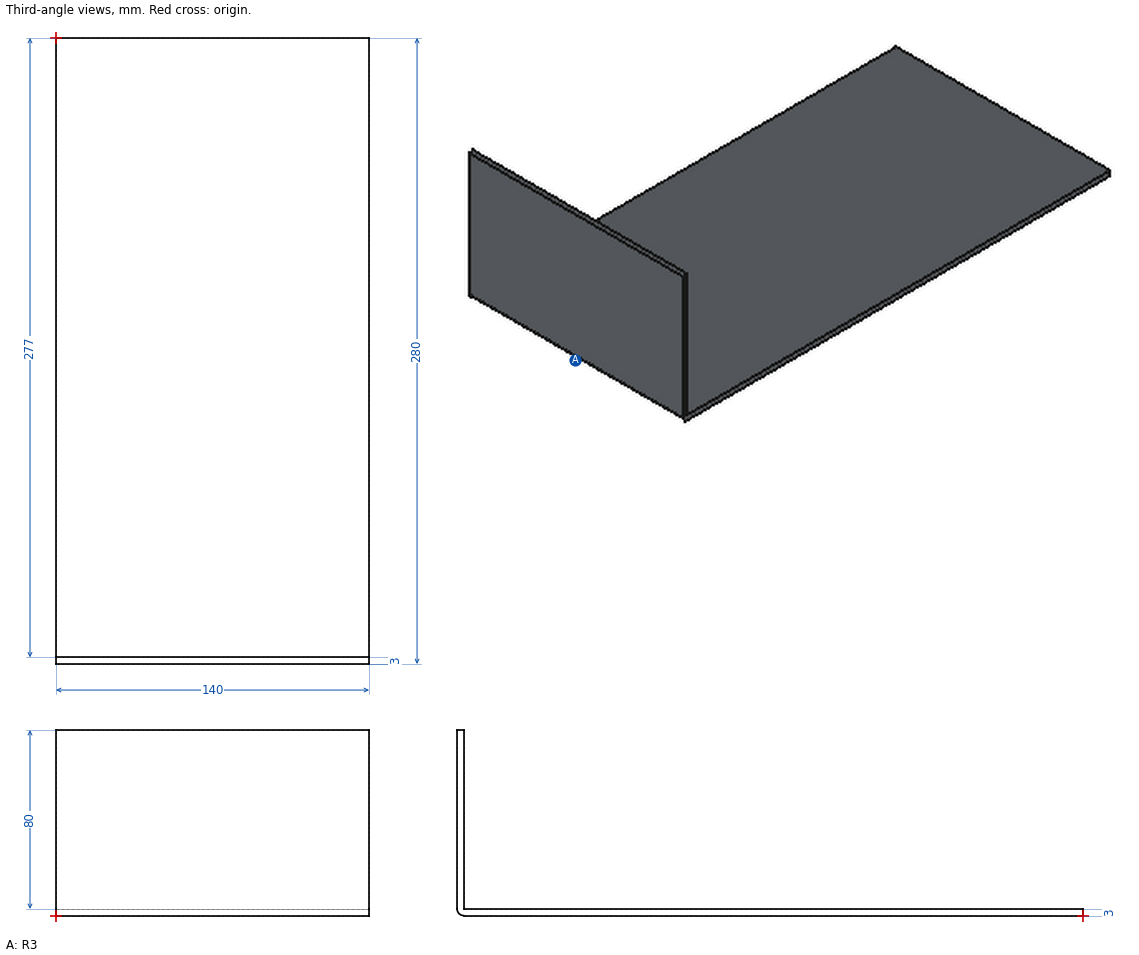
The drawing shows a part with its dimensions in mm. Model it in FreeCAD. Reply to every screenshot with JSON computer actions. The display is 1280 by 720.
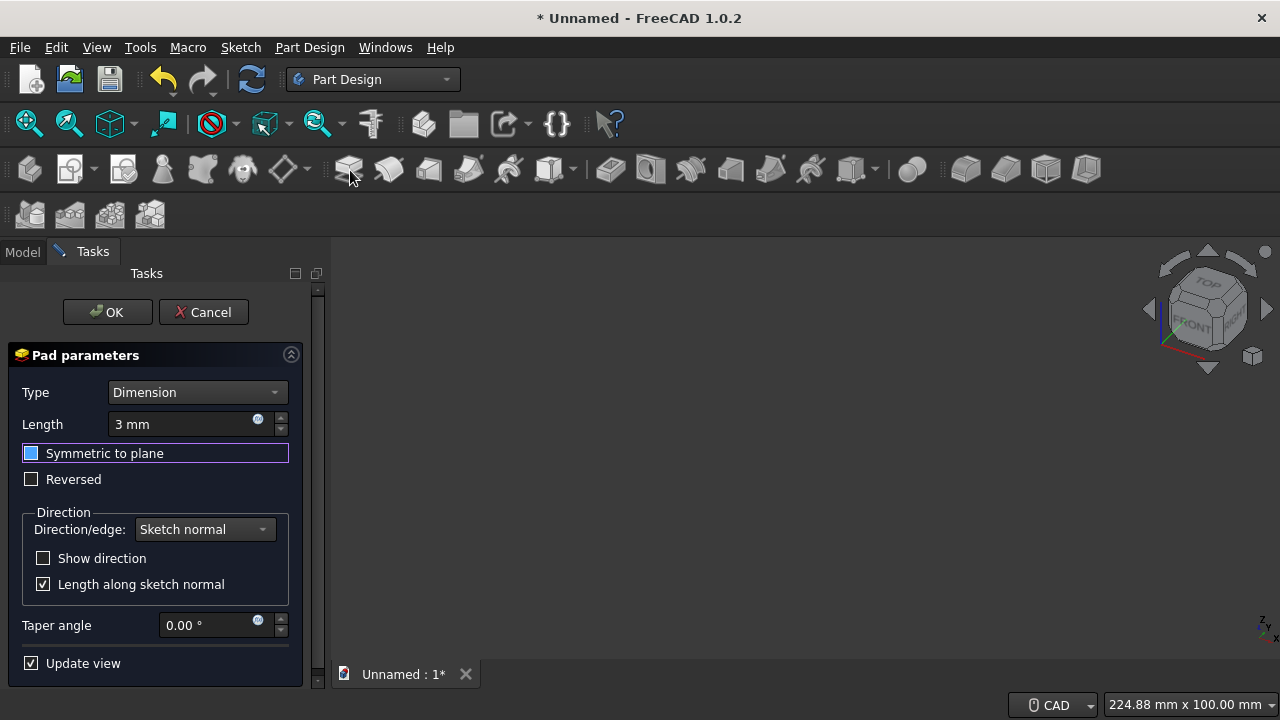
{"action": "left_click", "coordinate": [108, 312]}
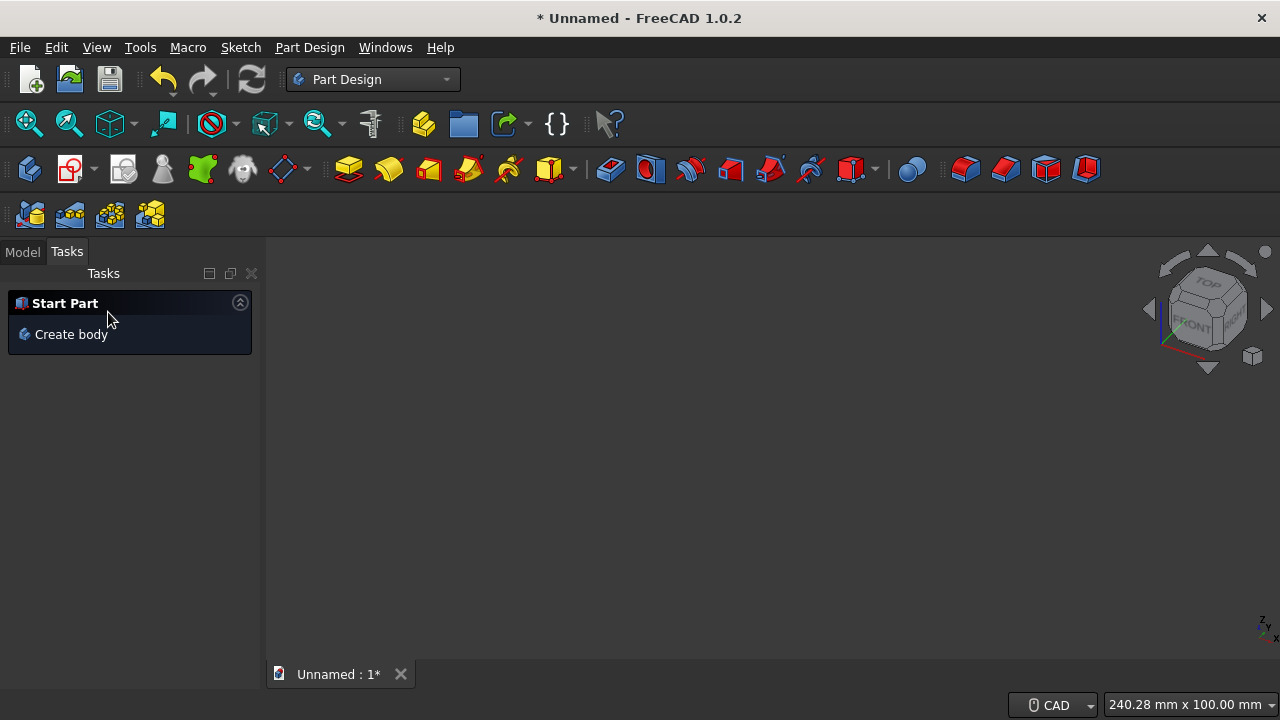
{"action": "key", "text": "v f"}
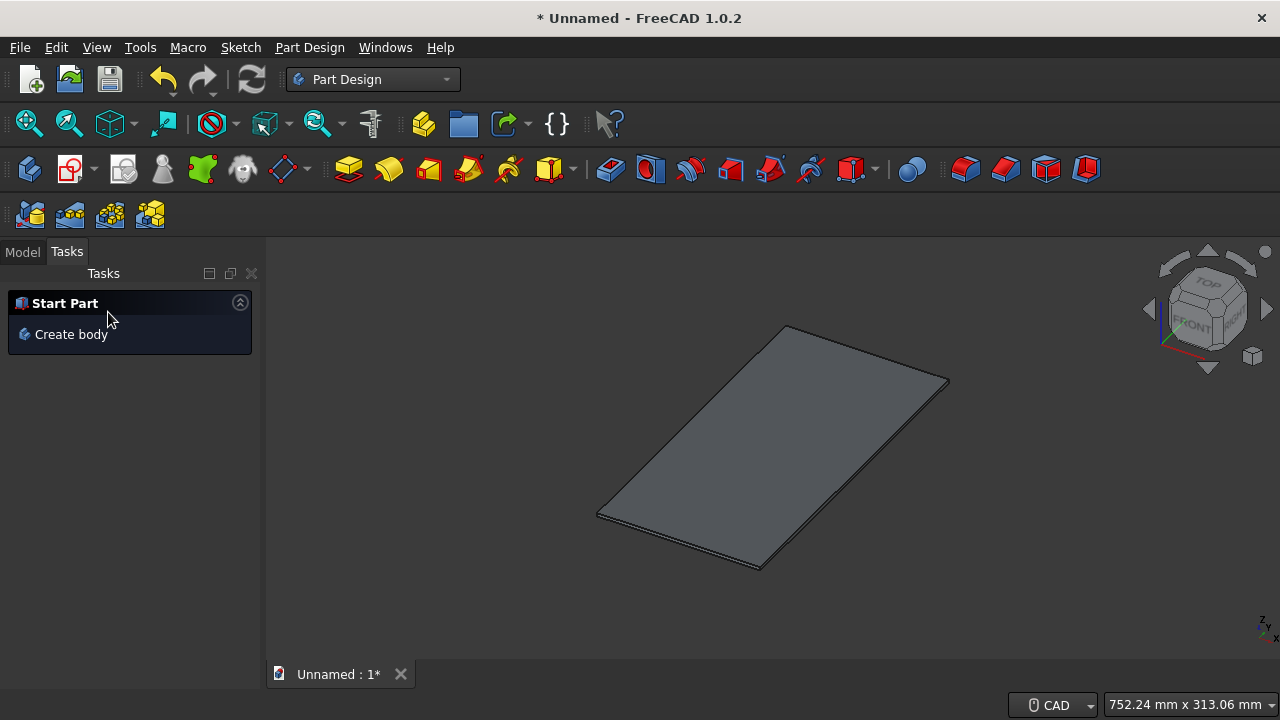
{"action": "left_click", "coordinate": [800, 419]}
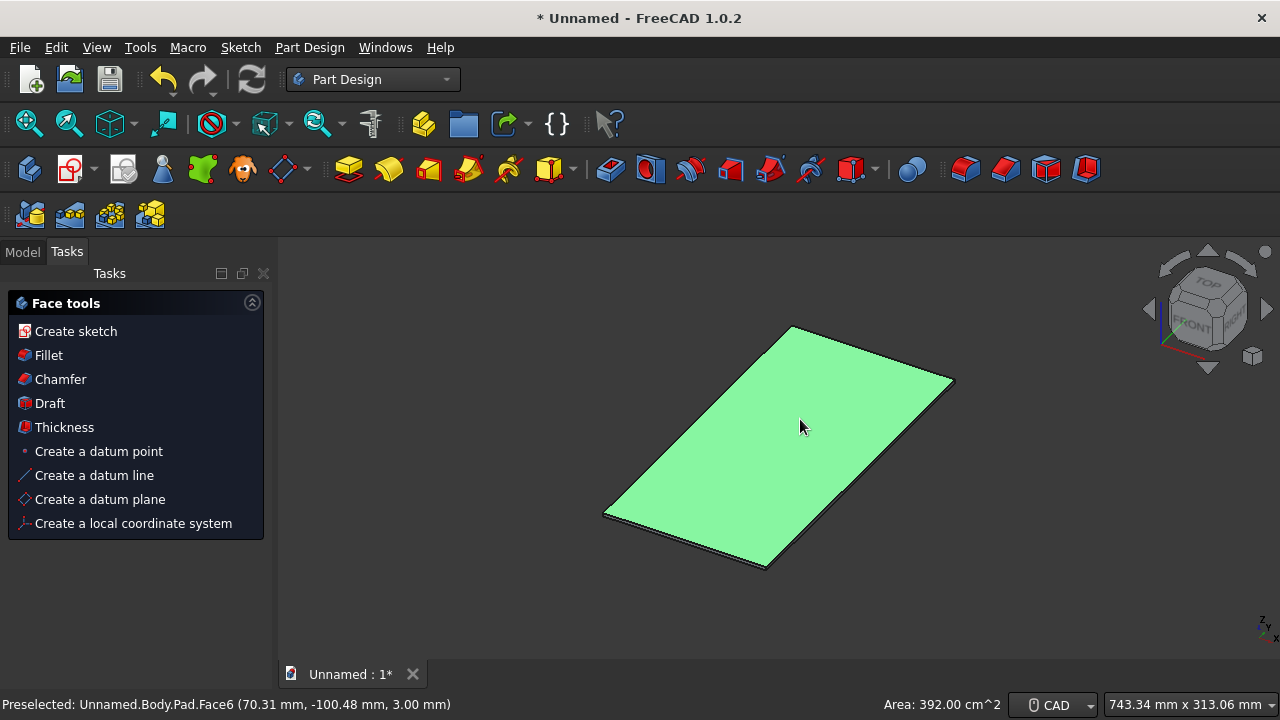
{"action": "left_click", "coordinate": [70, 170]}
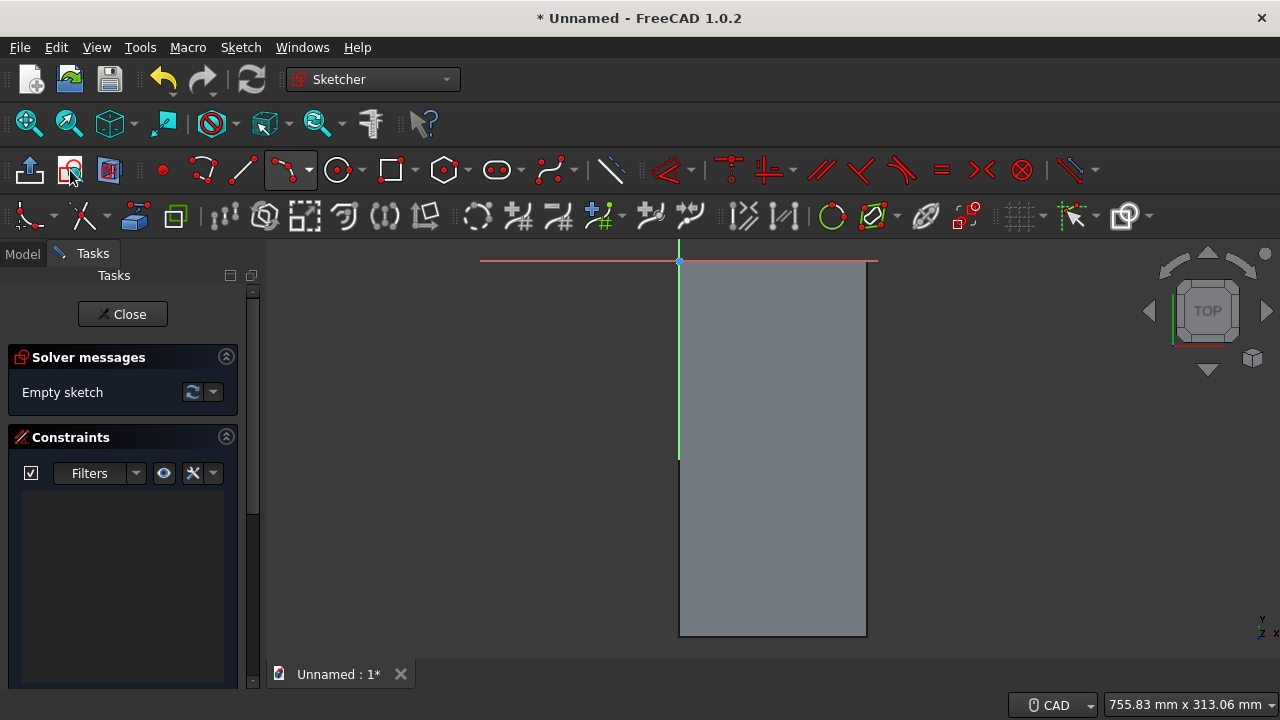
{"action": "scroll", "coordinate": [565, 449], "scroll_direction": "down", "scroll_amount": 2}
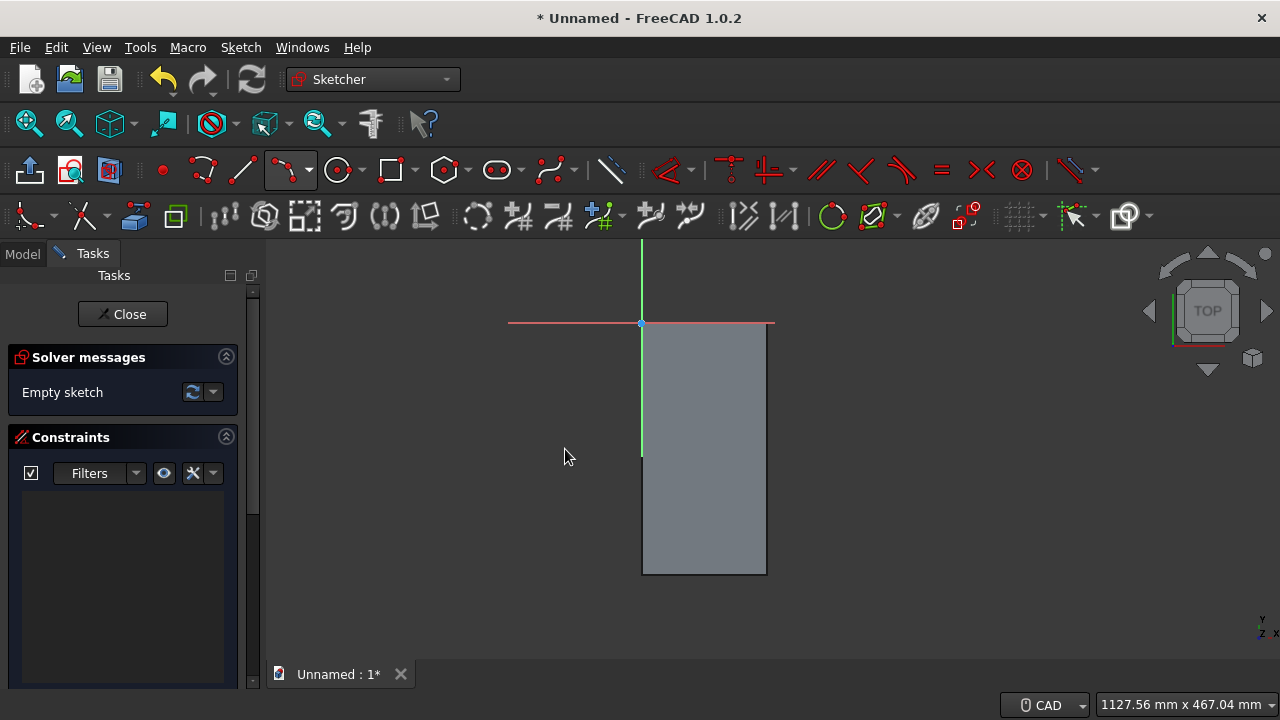
{"action": "left_click", "coordinate": [392, 170]}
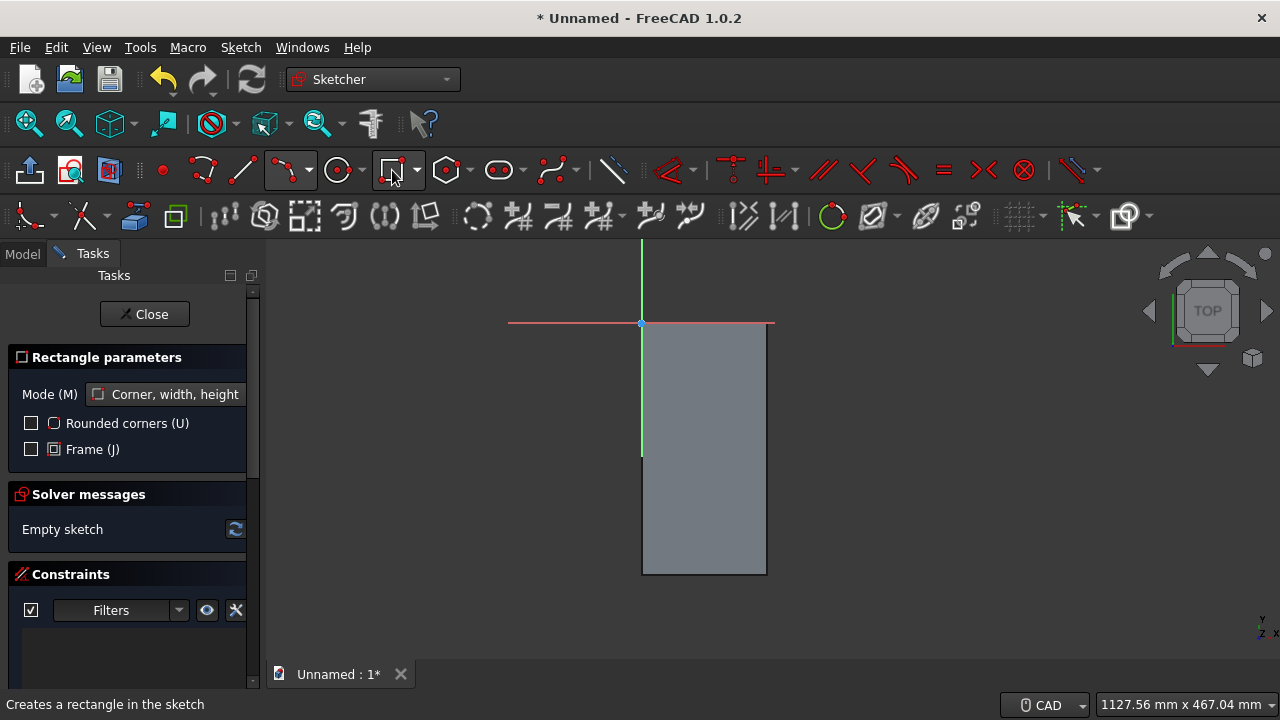
{"action": "scroll", "coordinate": [642, 572], "scroll_direction": "up", "scroll_amount": 9}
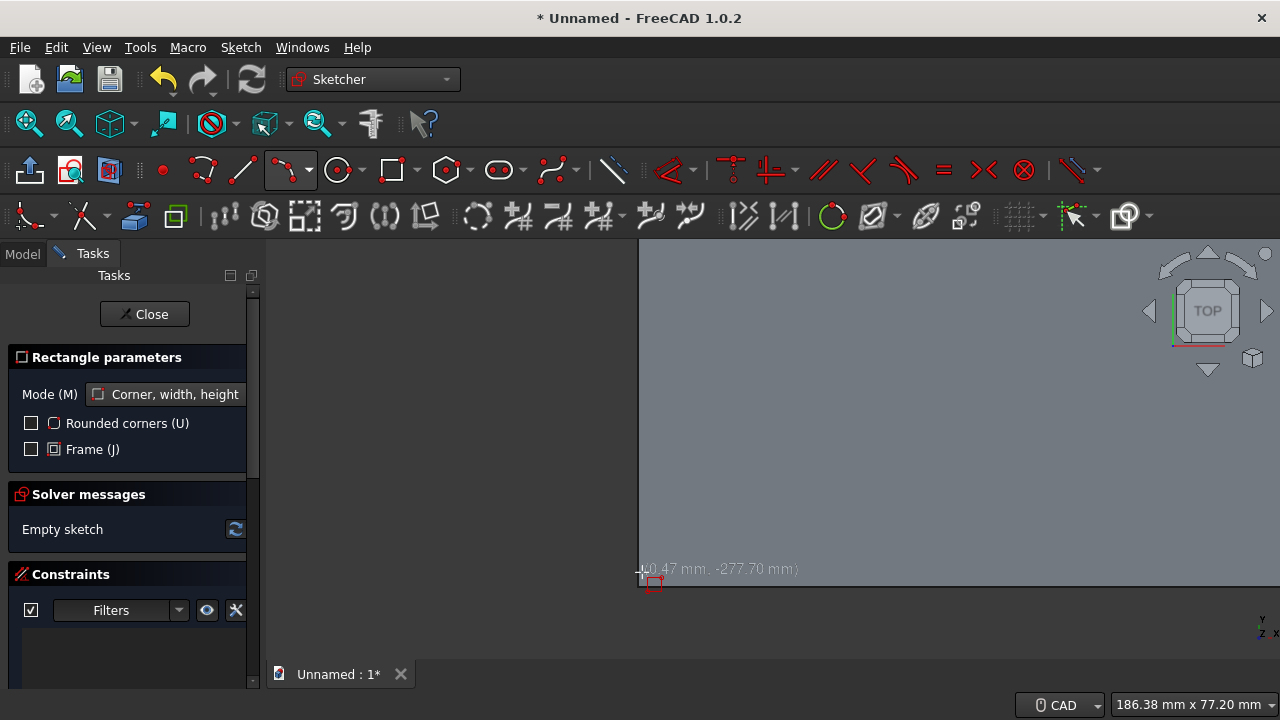
{"action": "scroll", "coordinate": [642, 573], "scroll_direction": "down", "scroll_amount": 9}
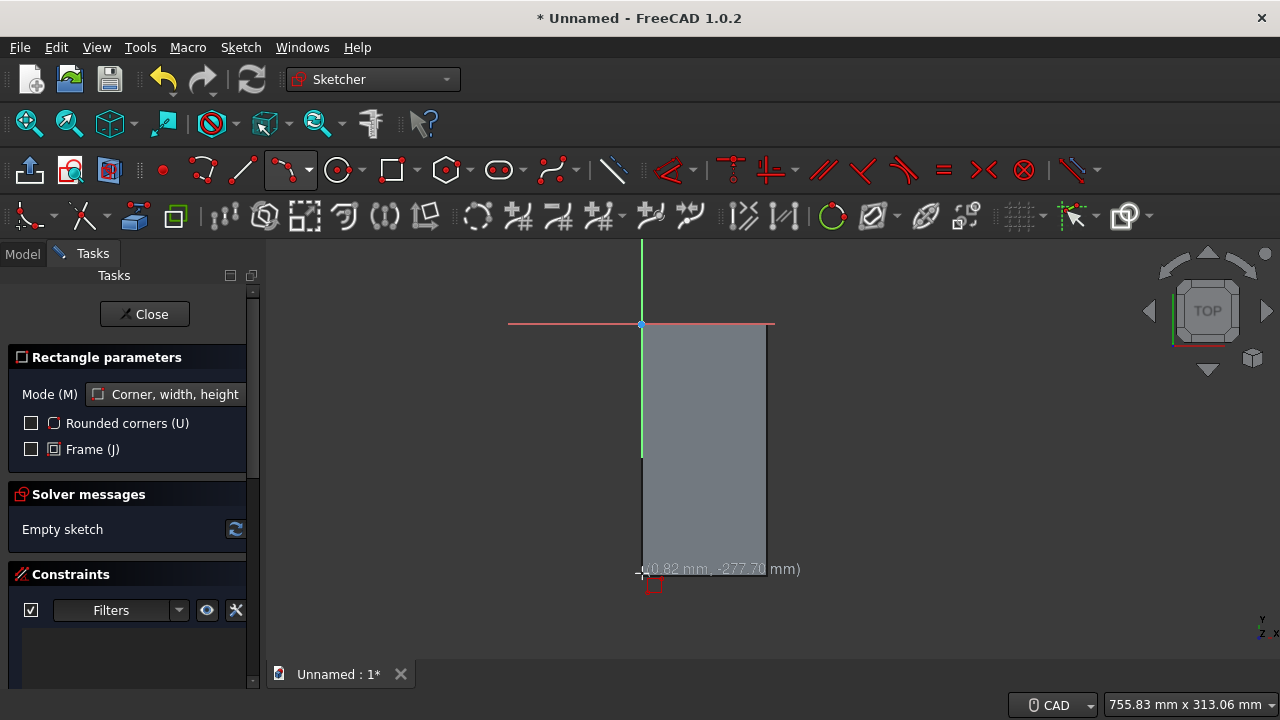
{"action": "left_click", "coordinate": [642, 573]}
{"action": "mouse_move", "coordinate": [767, 576]}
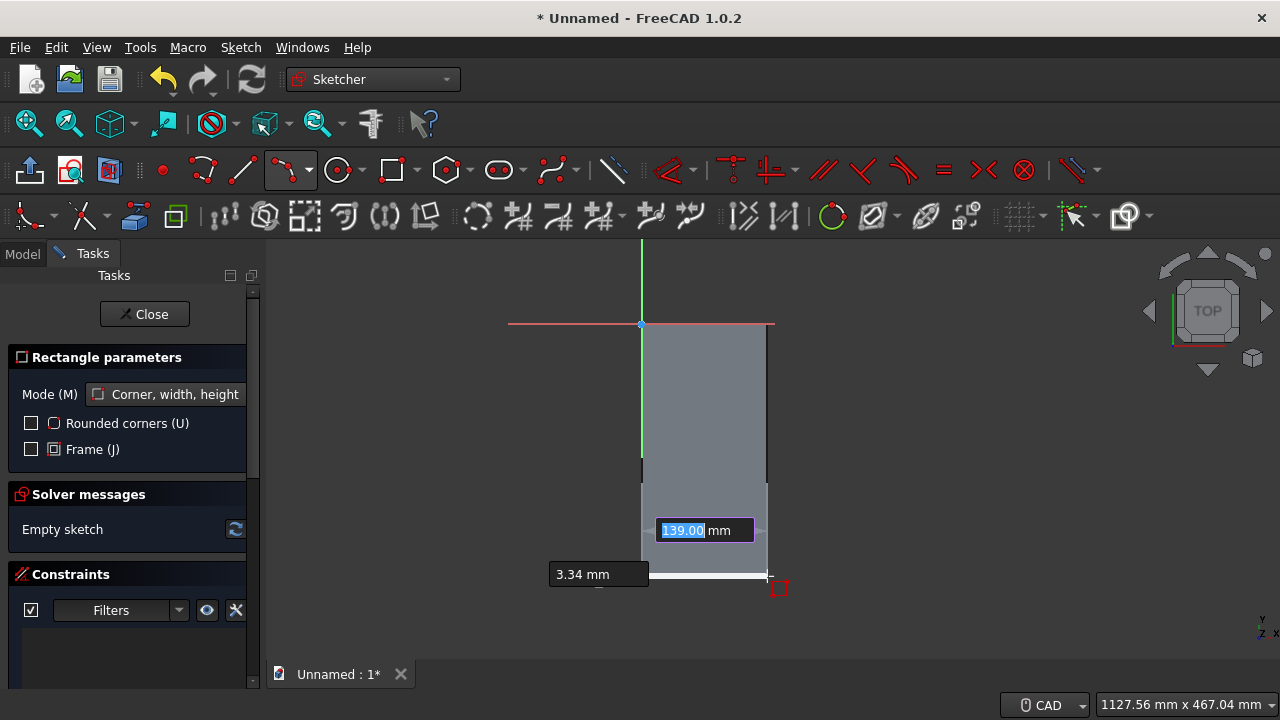
{"action": "type", "text": "140"}
{"action": "key", "text": "Tab"}
{"action": "type", "text": "3"}
{"action": "key", "text": "Return"}
{"action": "key", "text": "Escape"}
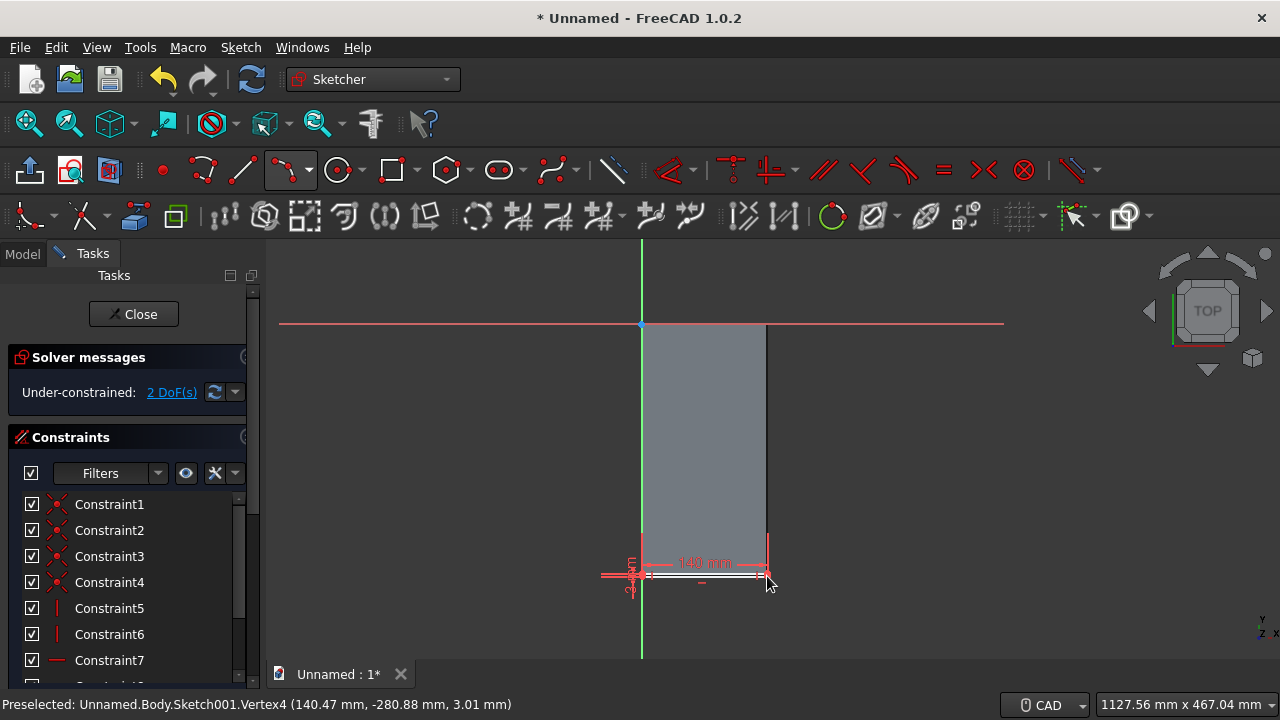
{"action": "scroll", "coordinate": [642, 574], "scroll_direction": "up", "scroll_amount": 8}